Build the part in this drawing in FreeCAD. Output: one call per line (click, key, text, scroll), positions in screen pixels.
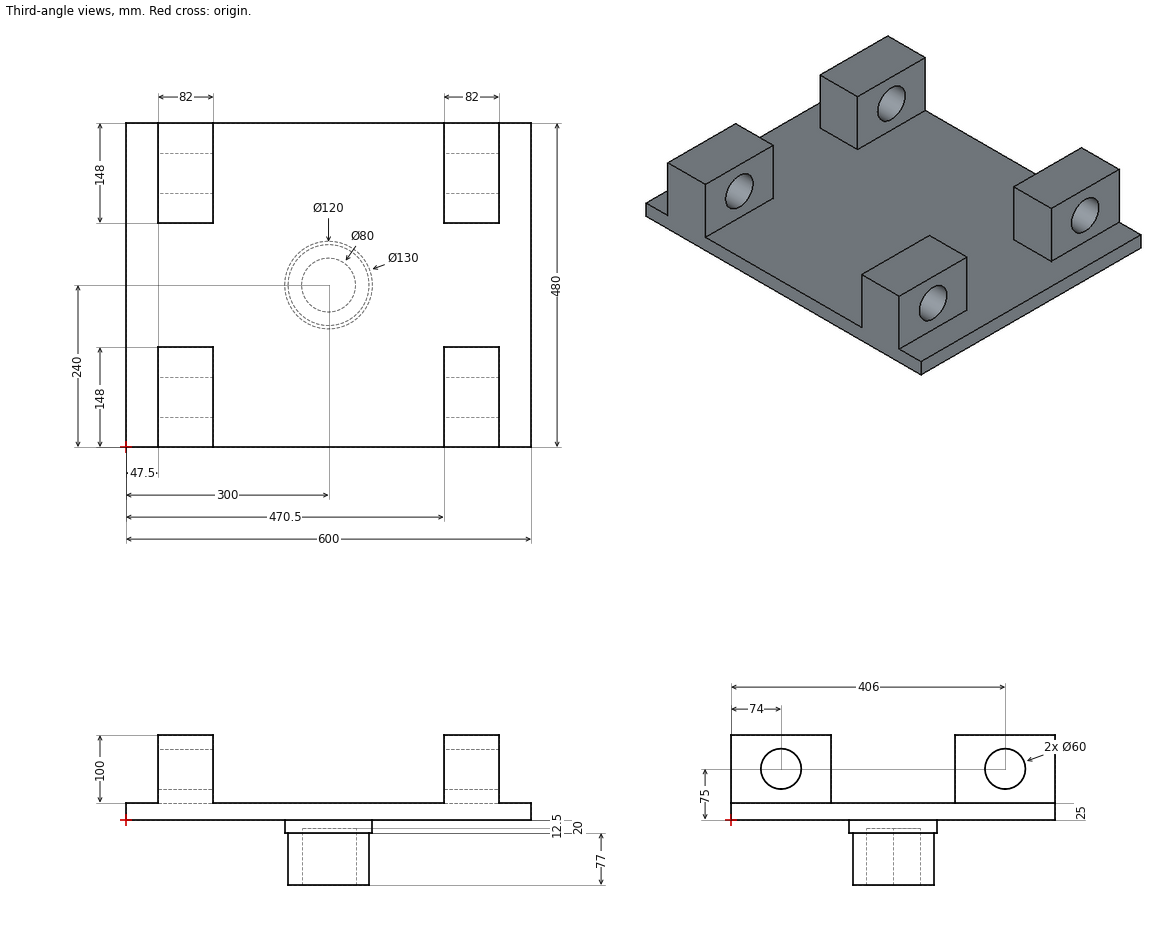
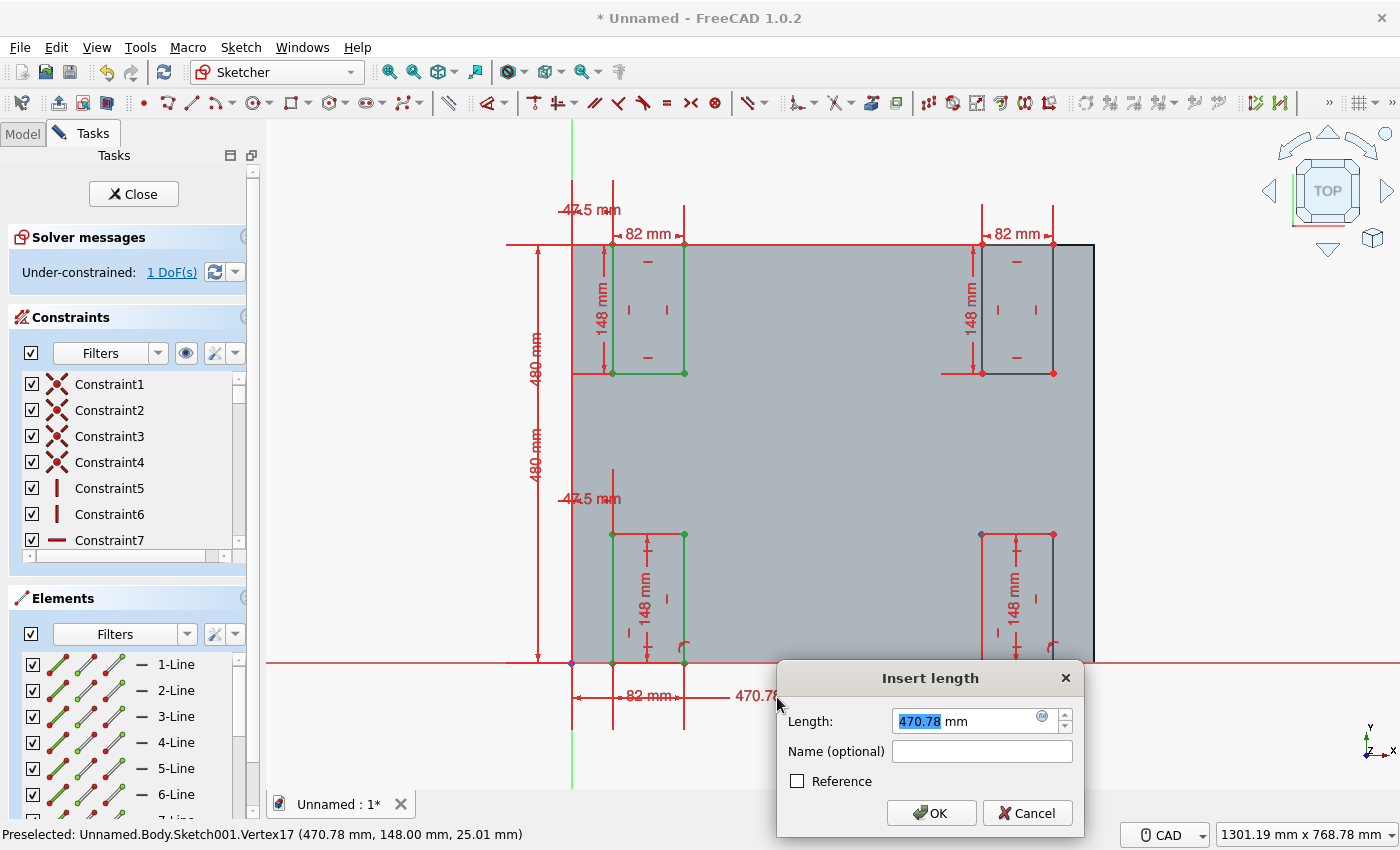
text(470.5)
key(Return)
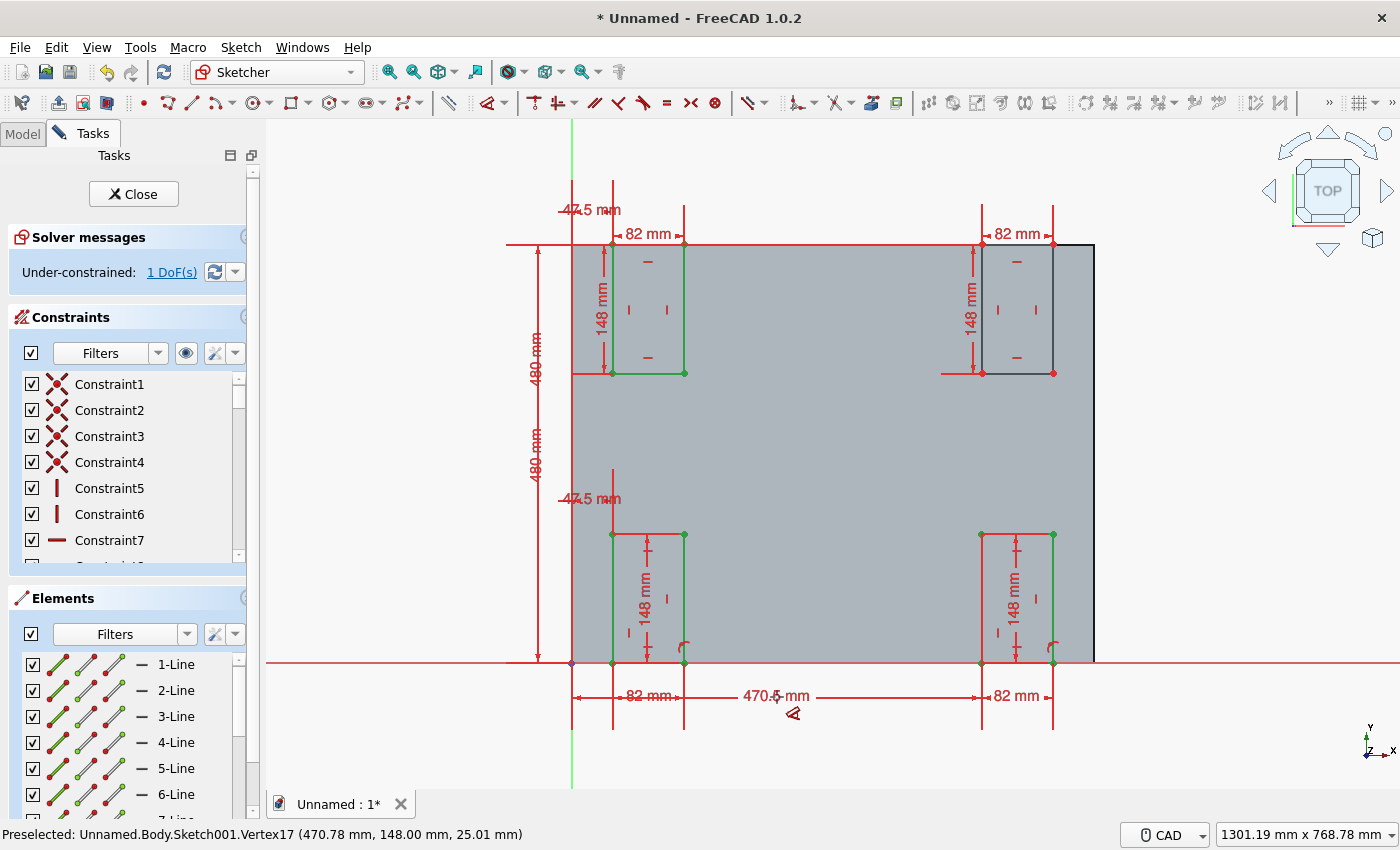
click(982, 245)
click(871, 697)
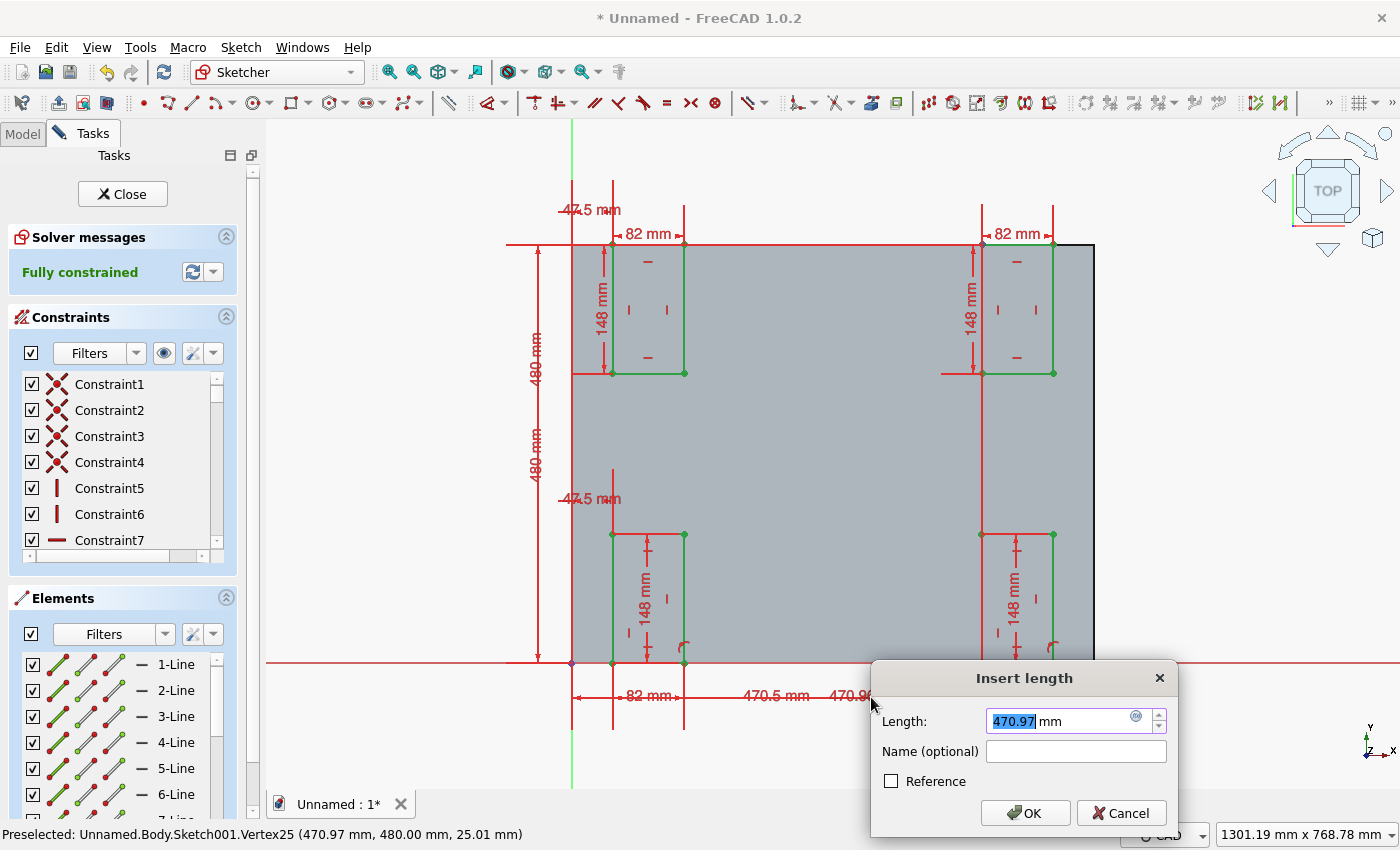
text(470.5)
key(Return)
key(Escape)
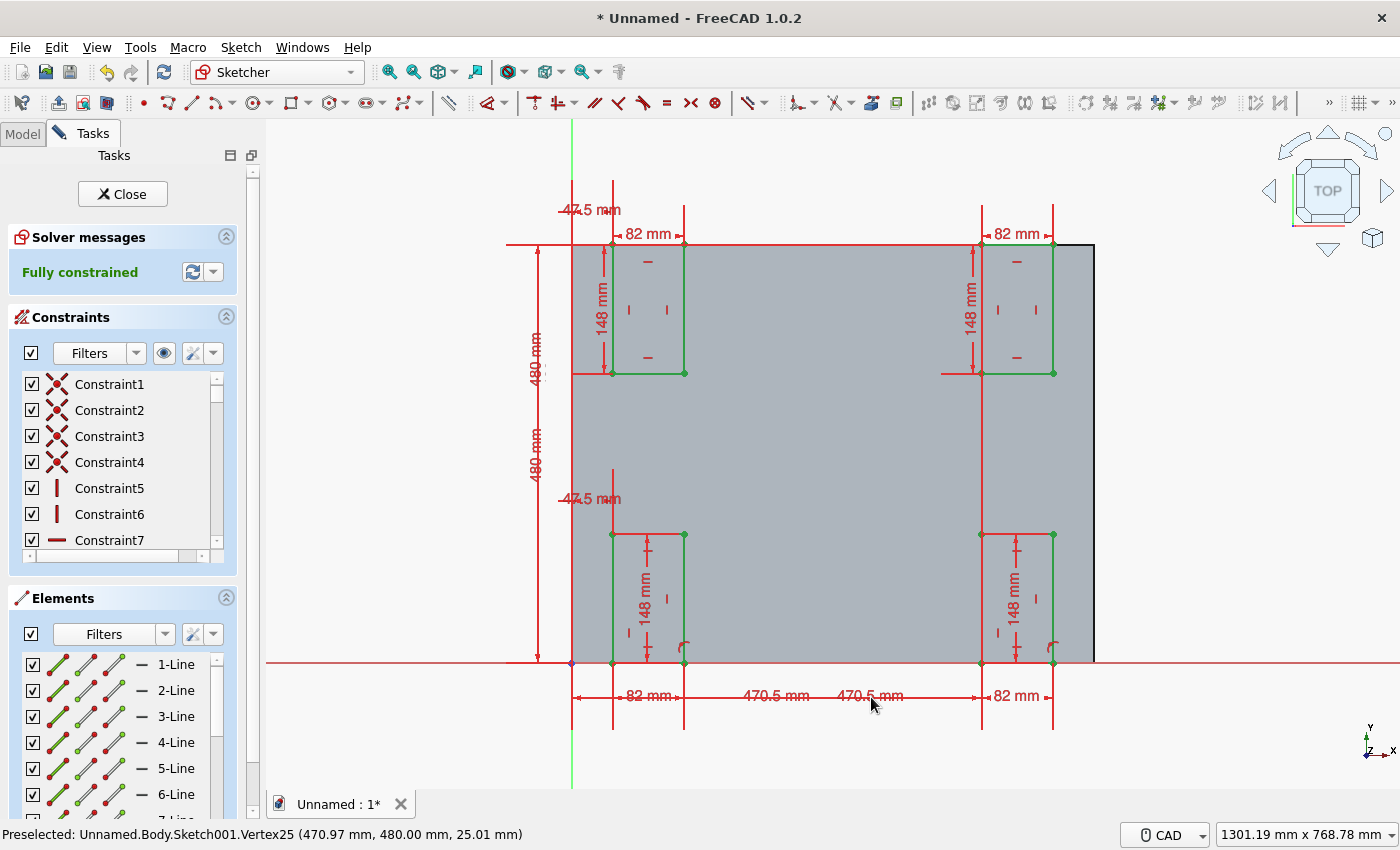
click(123, 194)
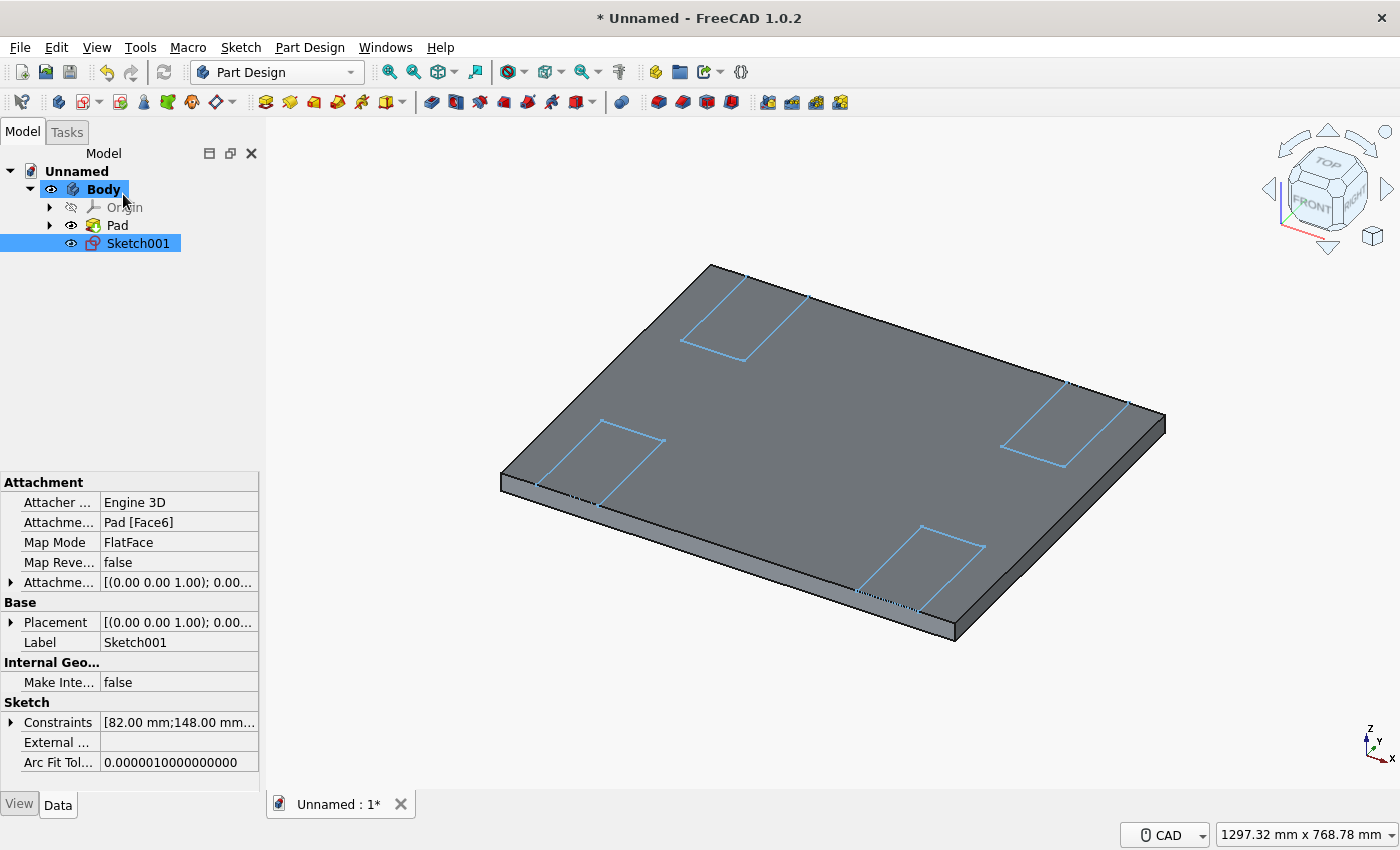
click(266, 102)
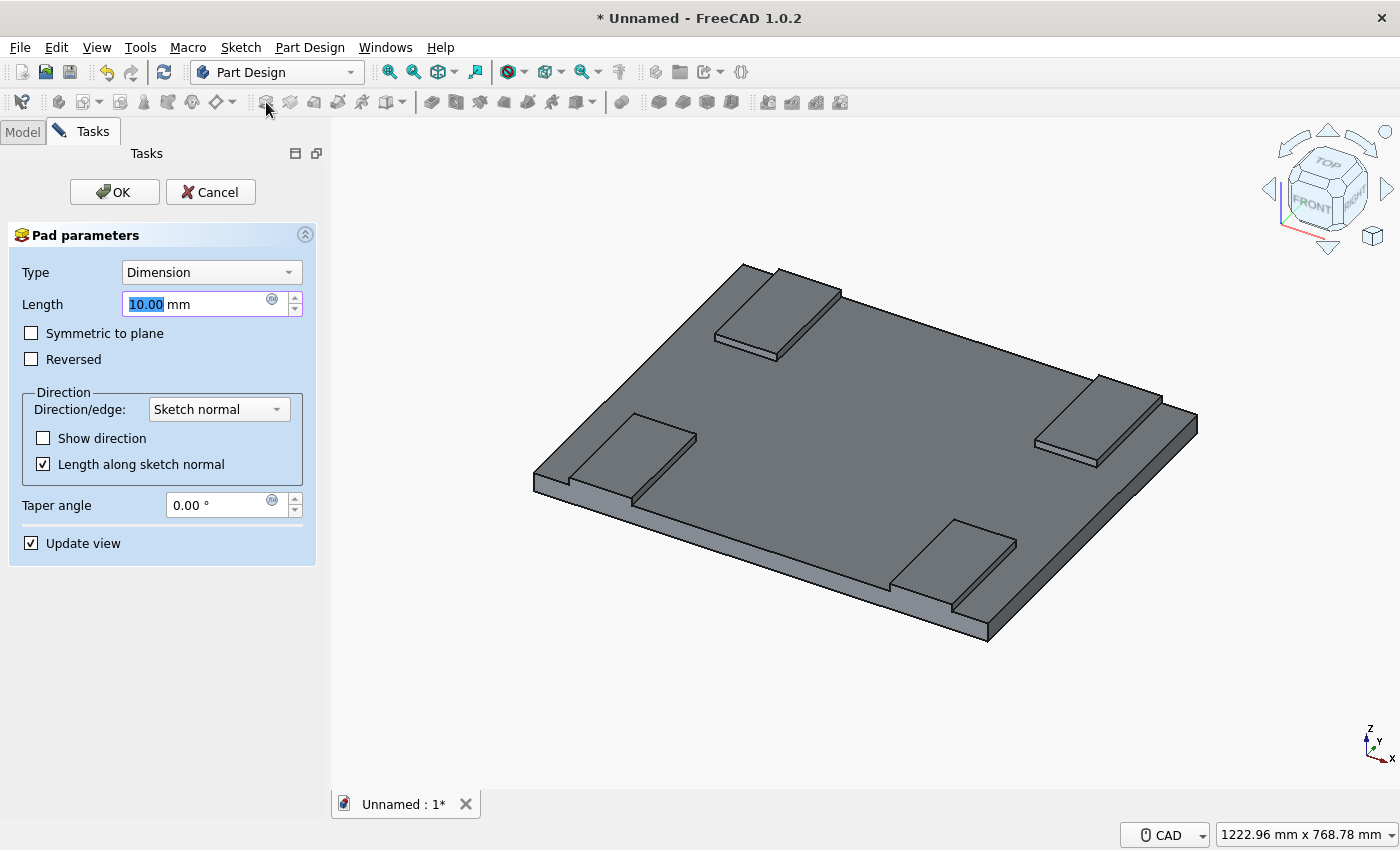
text(100)
key(Tab)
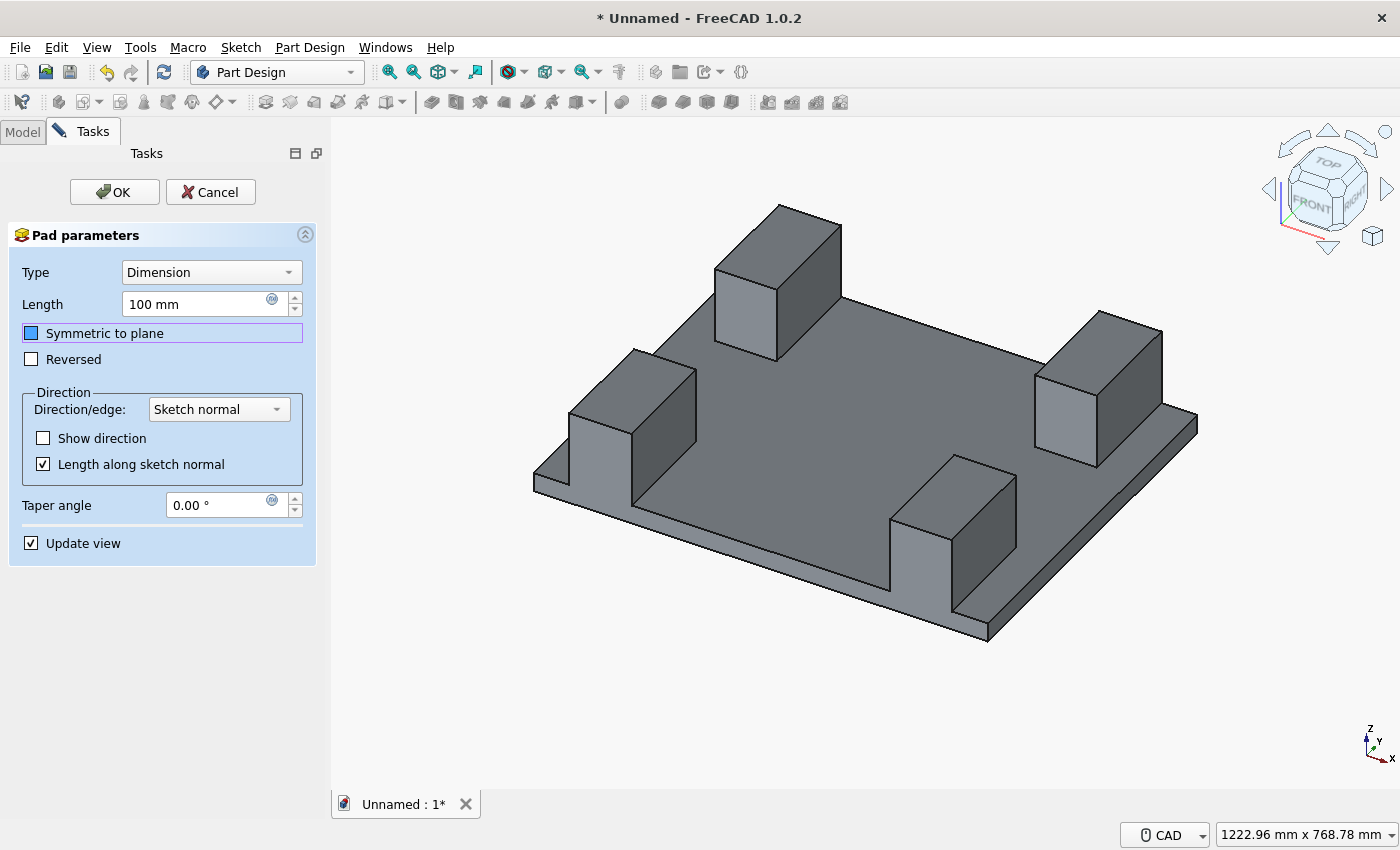
click(115, 192)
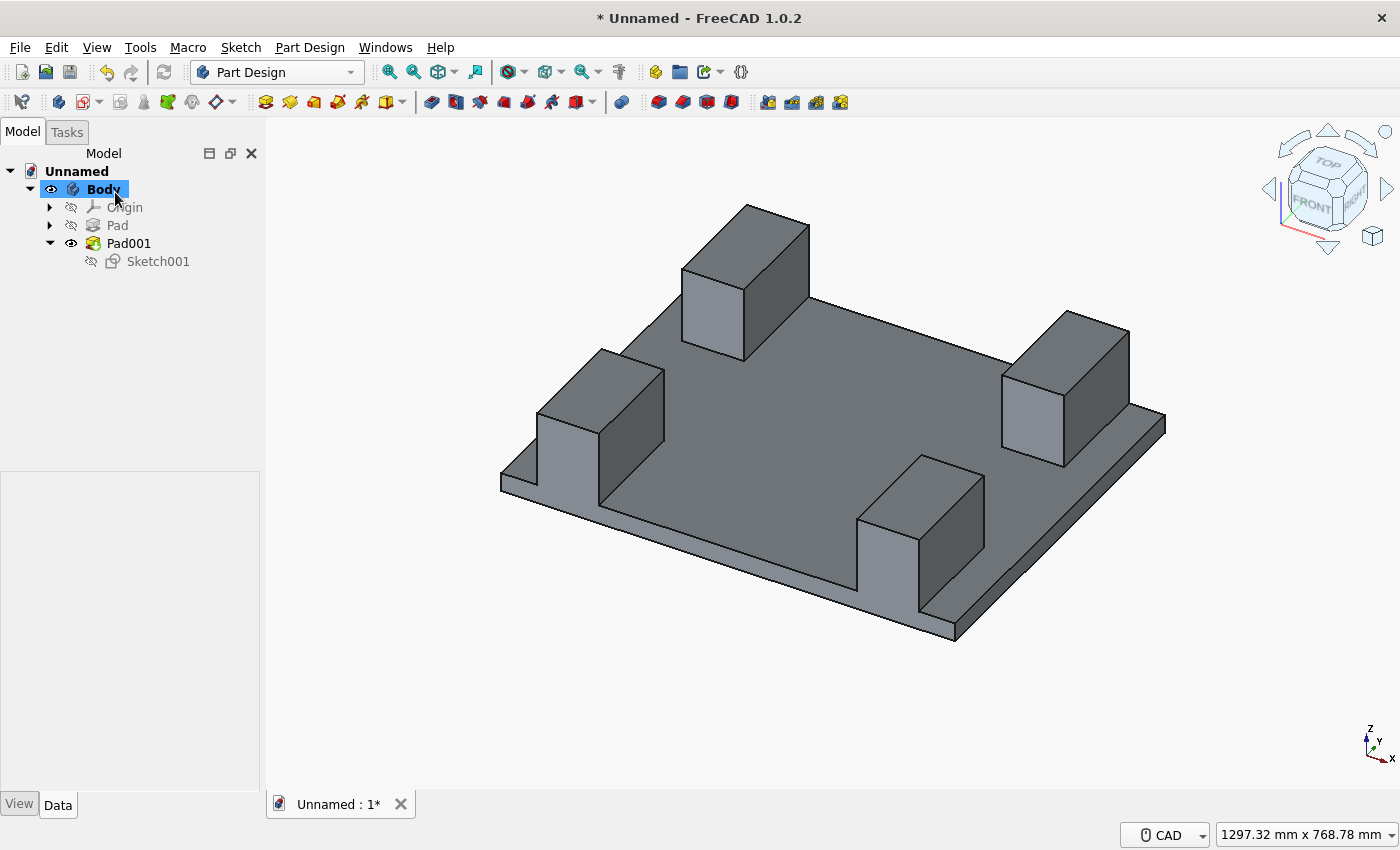
key(6)